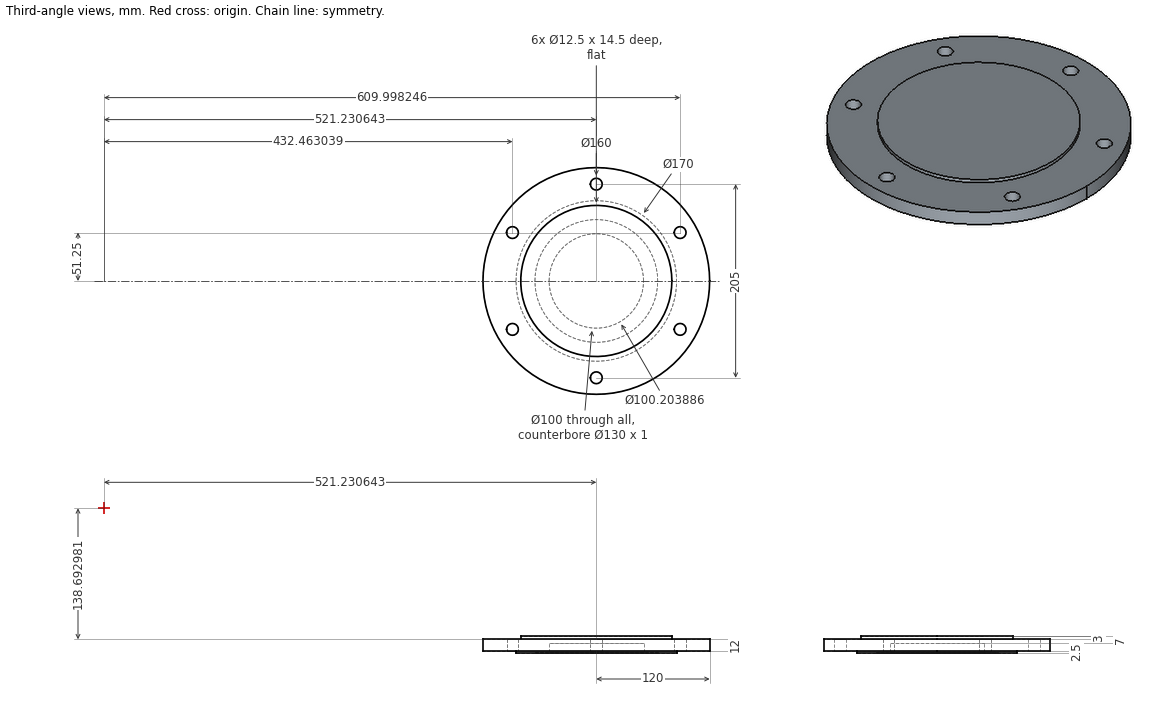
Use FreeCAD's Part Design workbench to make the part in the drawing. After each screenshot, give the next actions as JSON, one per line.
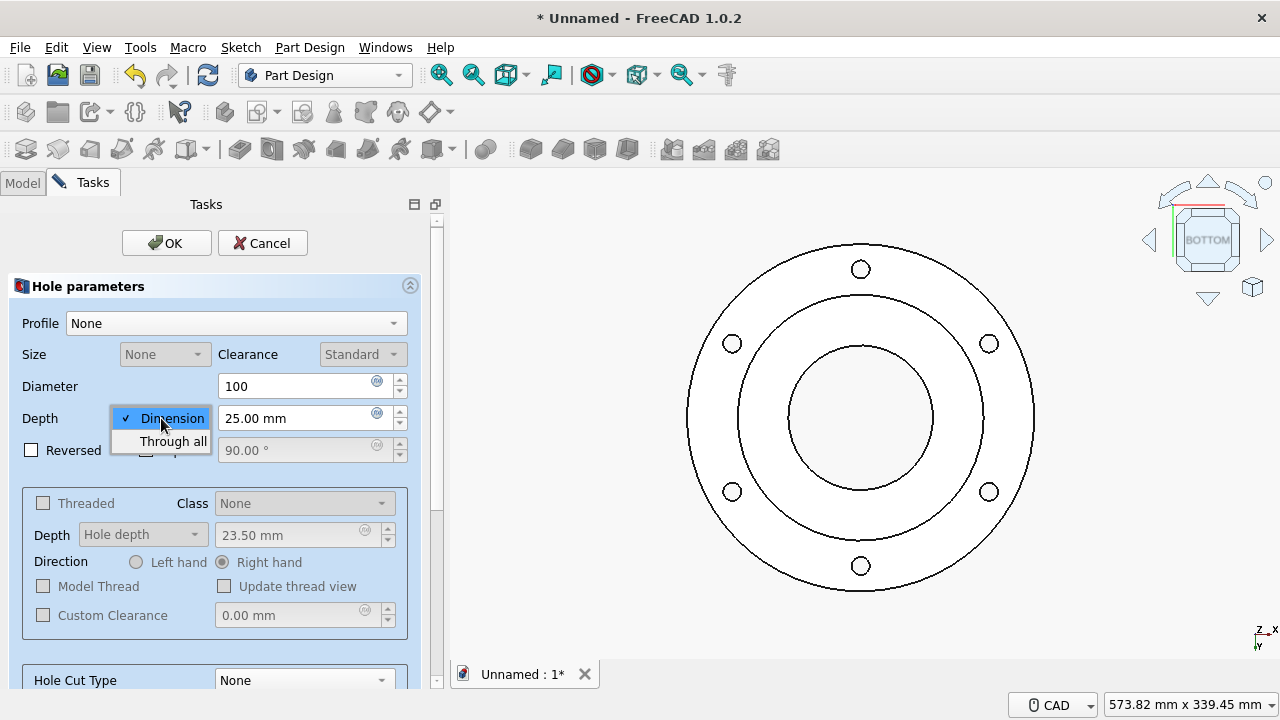
{"action": "left_click", "coordinate": [160, 442]}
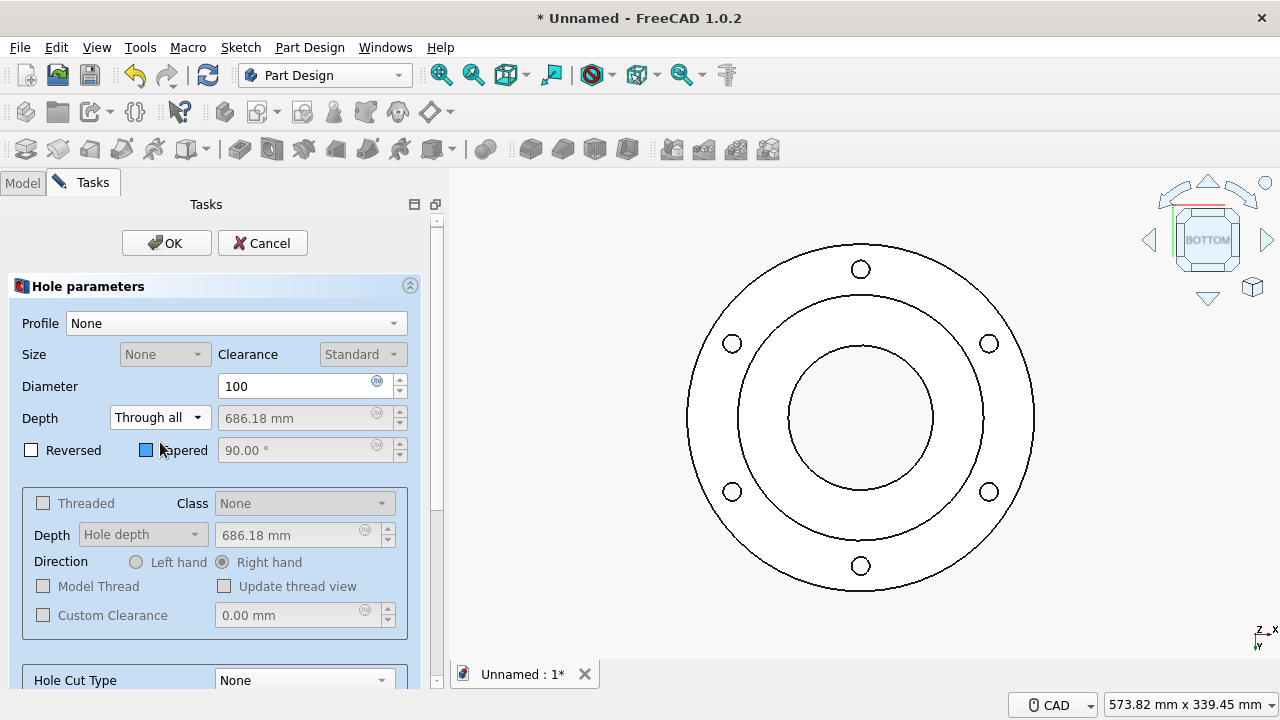
{"action": "scroll", "coordinate": [437, 451], "scroll_direction": "down", "scroll_amount": 2}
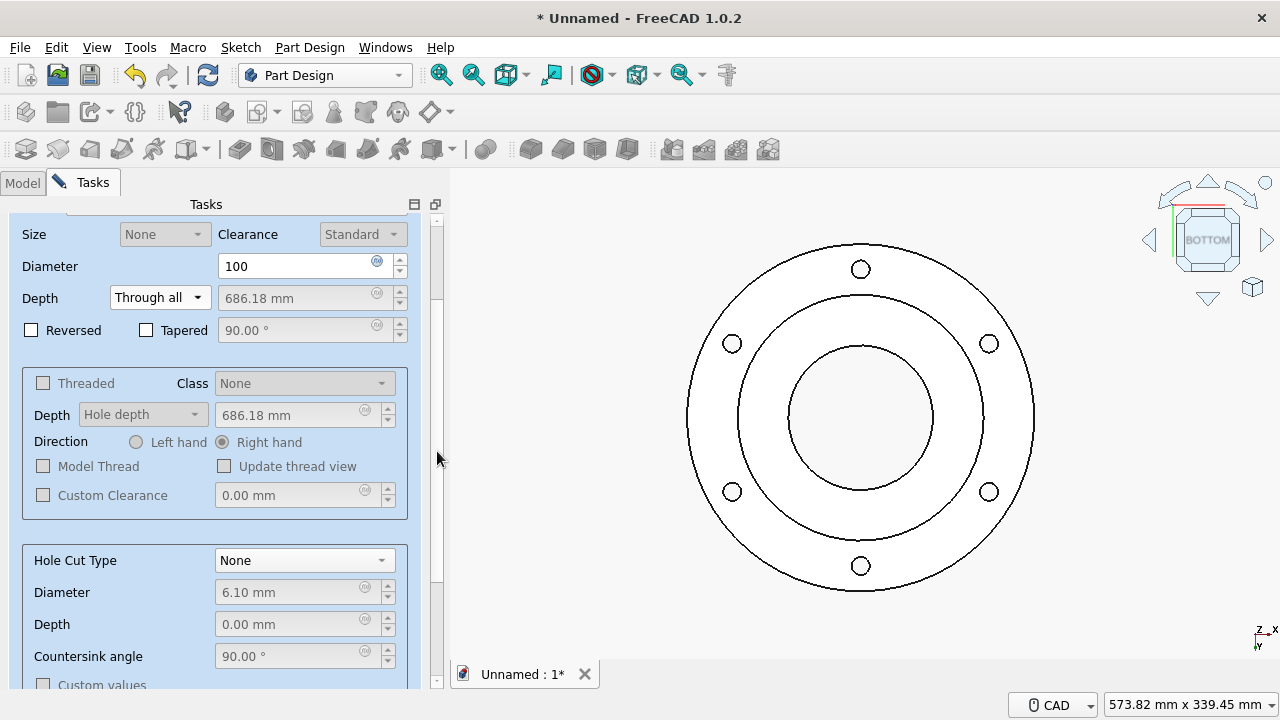
{"action": "left_click", "coordinate": [306, 560]}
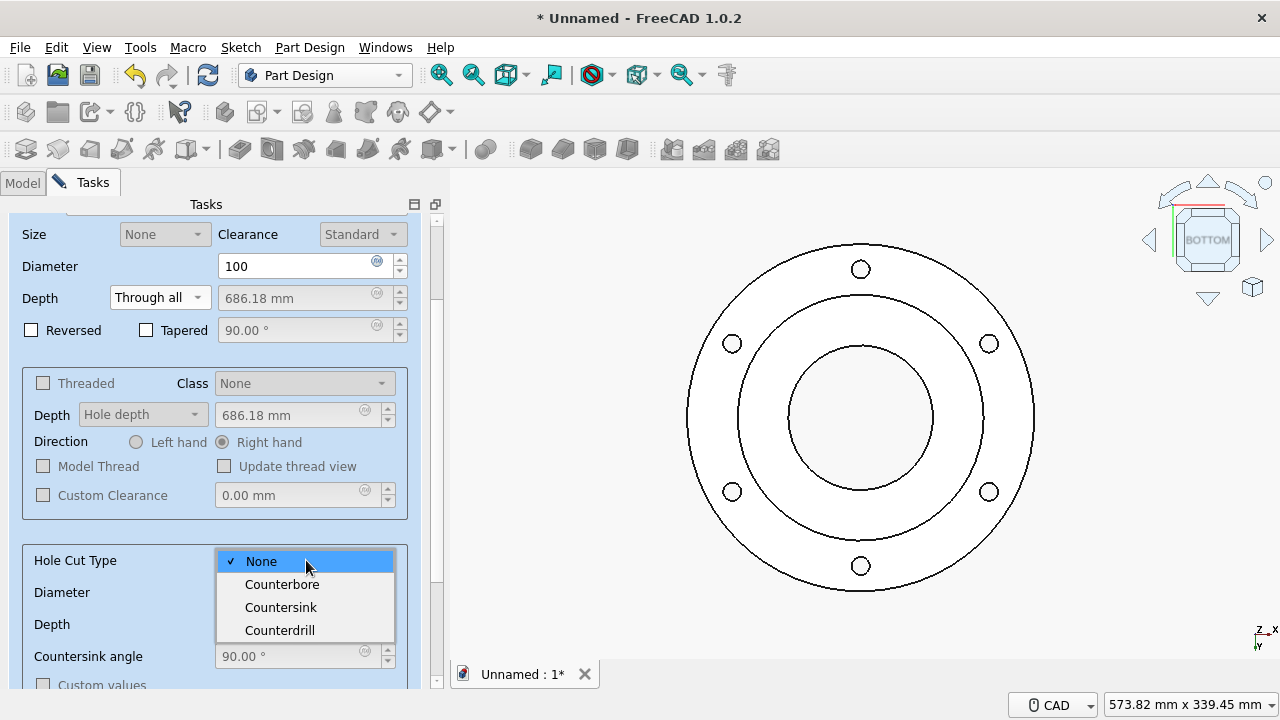
{"action": "left_click", "coordinate": [304, 584]}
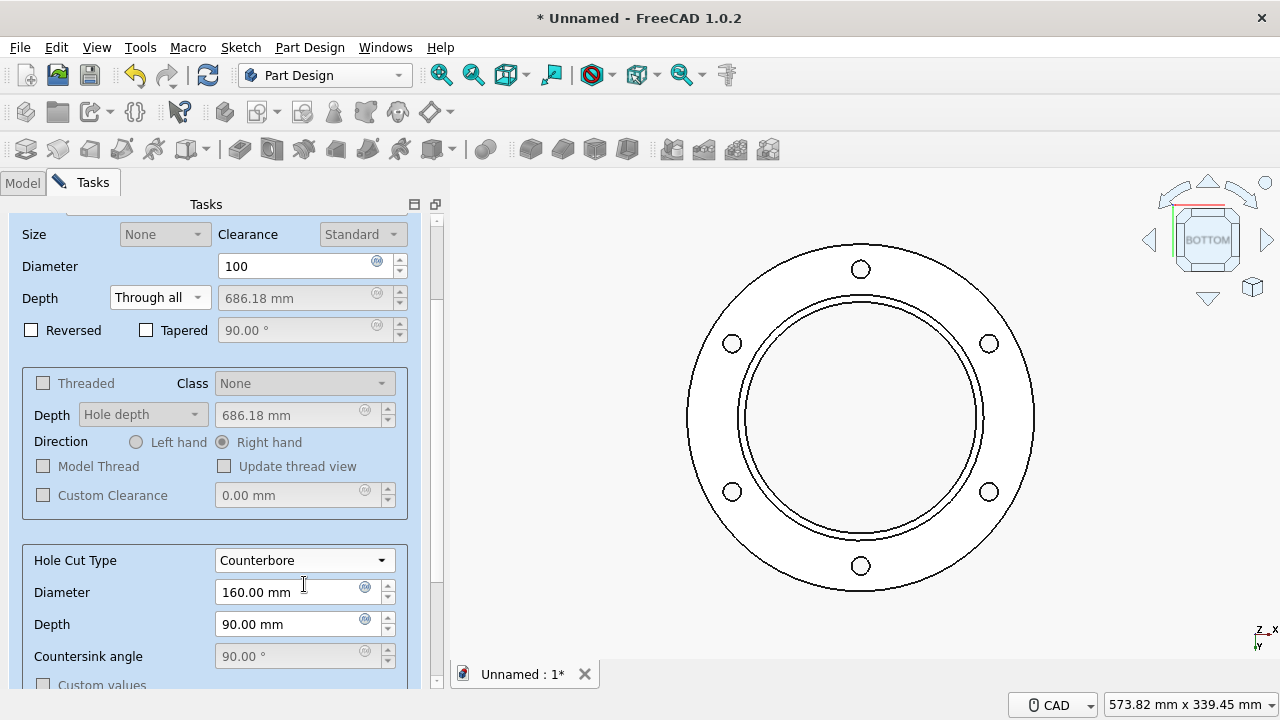
{"action": "triple_click", "coordinate": [298, 592]}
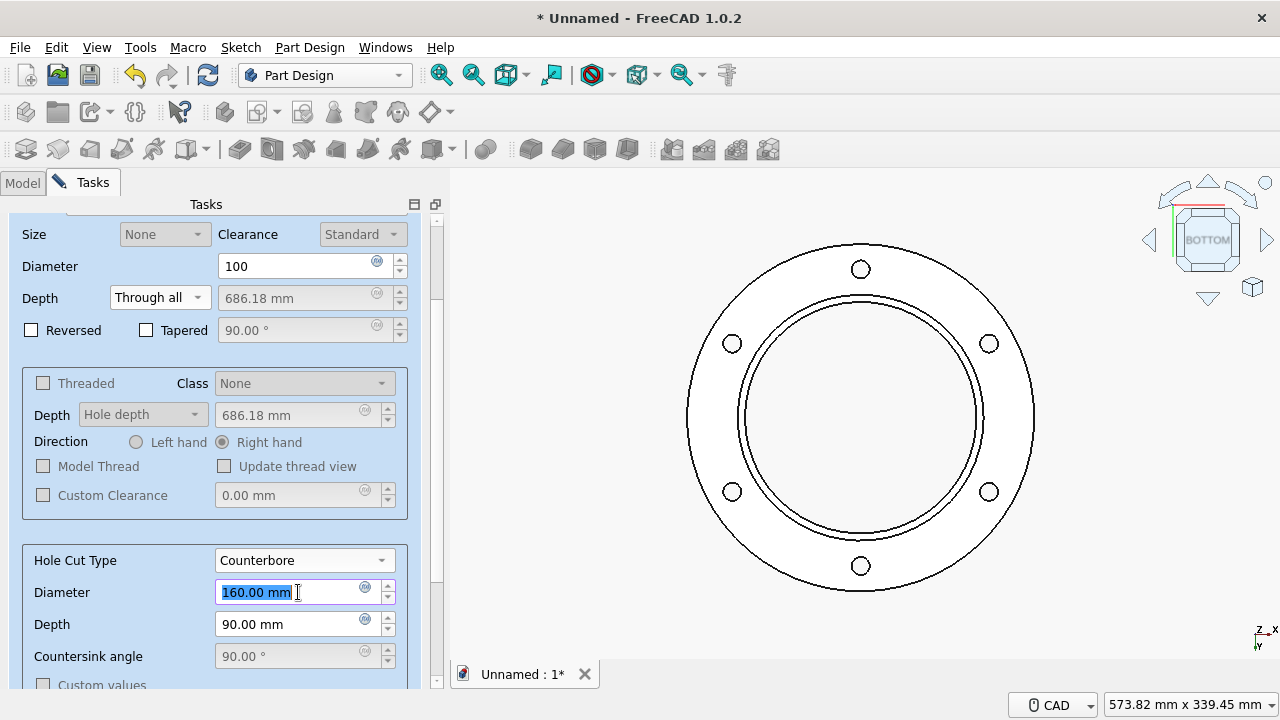
{"action": "type", "text": "130"}
{"action": "key", "text": "Tab"}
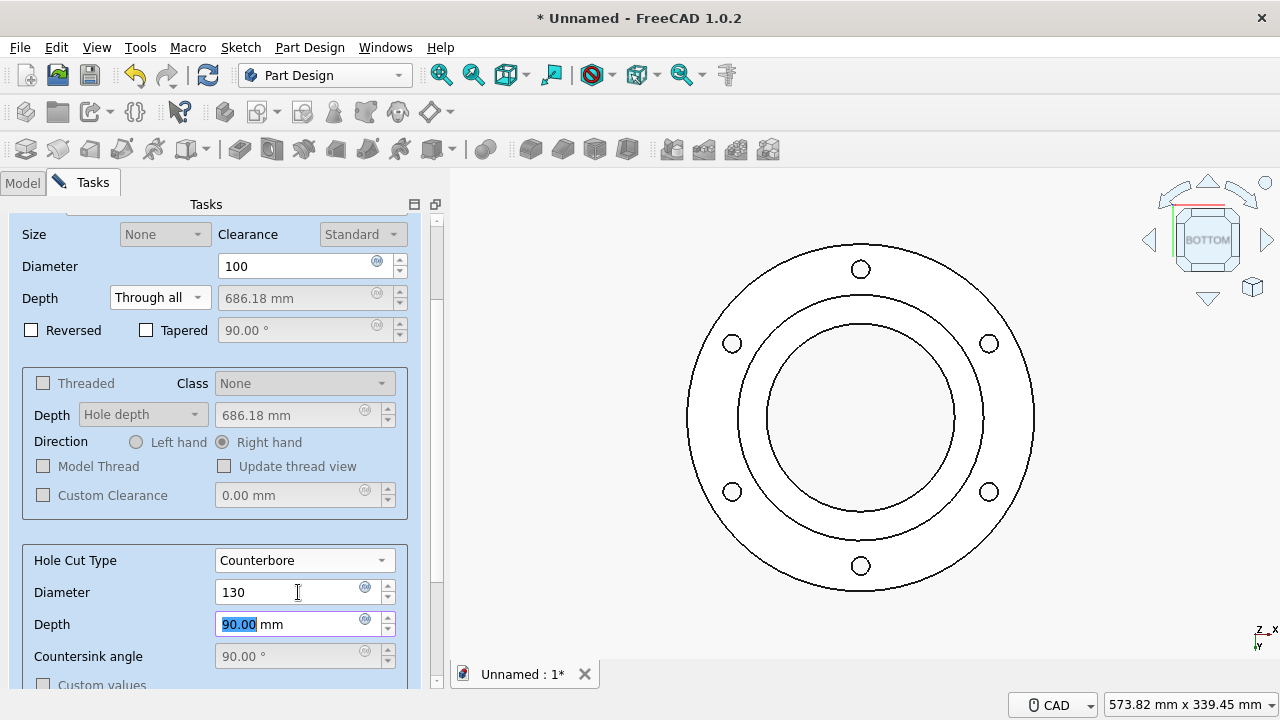
{"action": "type", "text": "1"}
{"action": "key", "text": "Tab"}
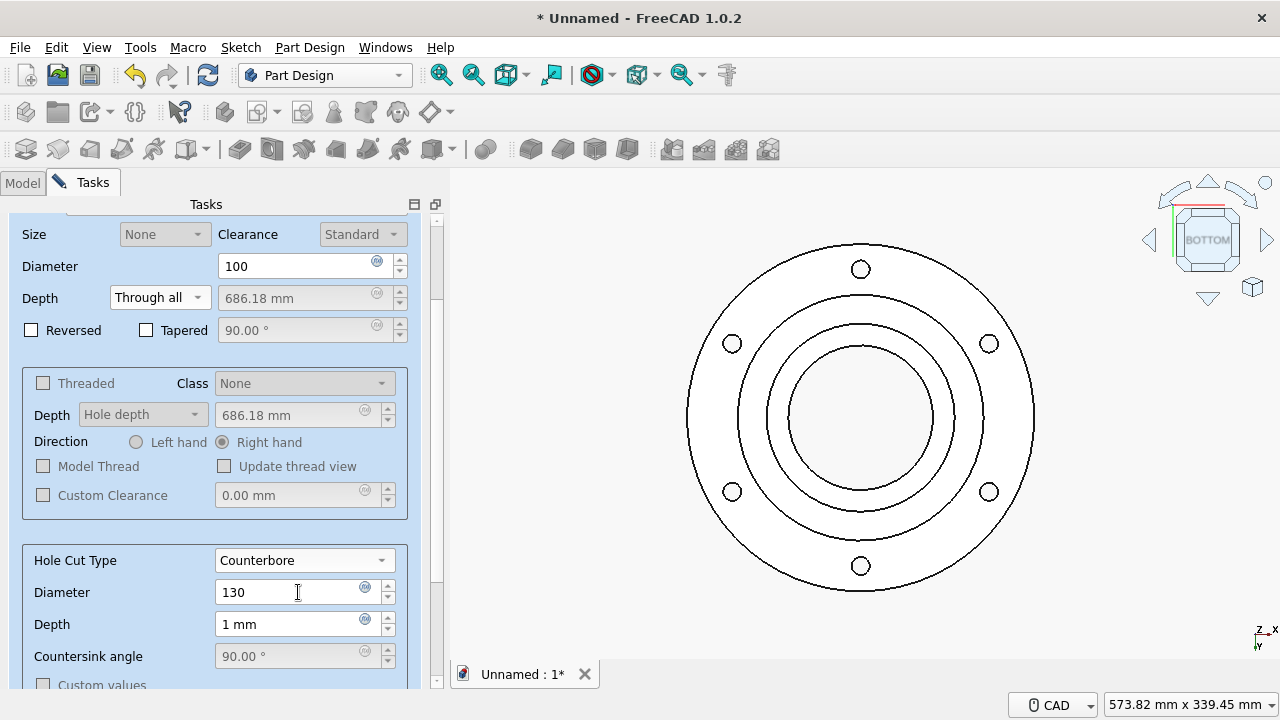
{"action": "scroll", "coordinate": [437, 451], "scroll_direction": "up", "scroll_amount": 3}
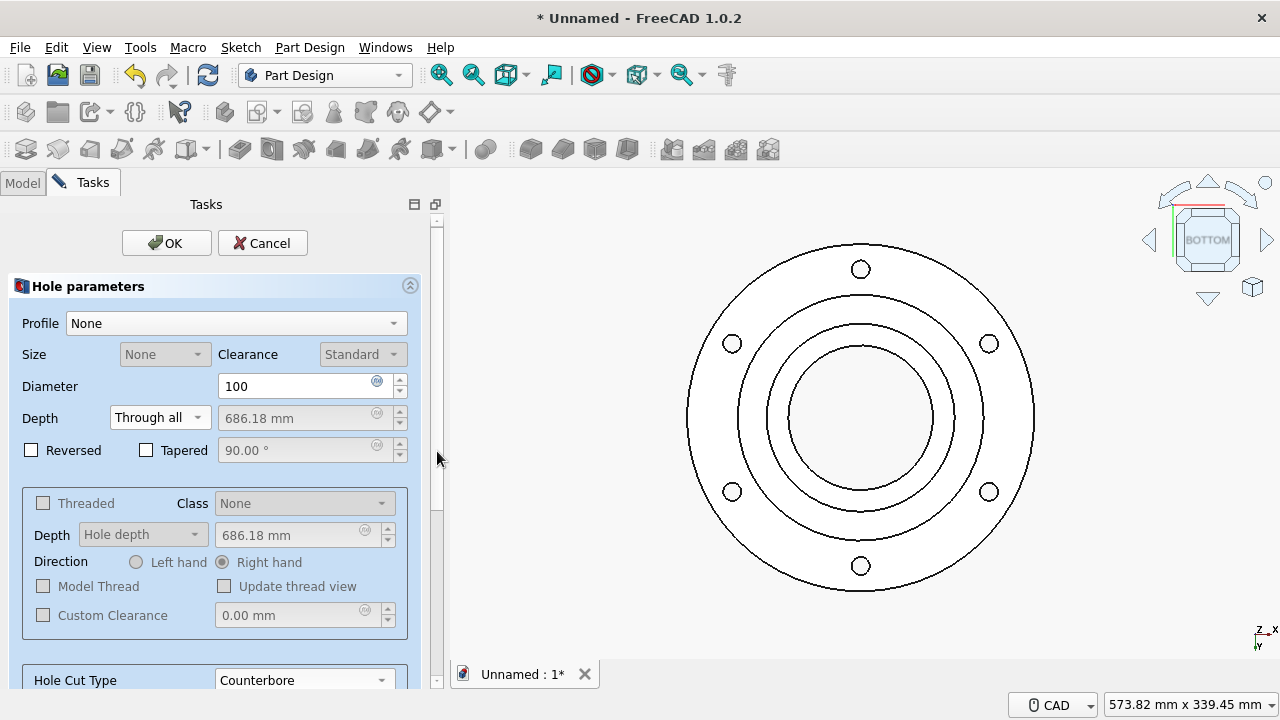
{"action": "left_click", "coordinate": [167, 243]}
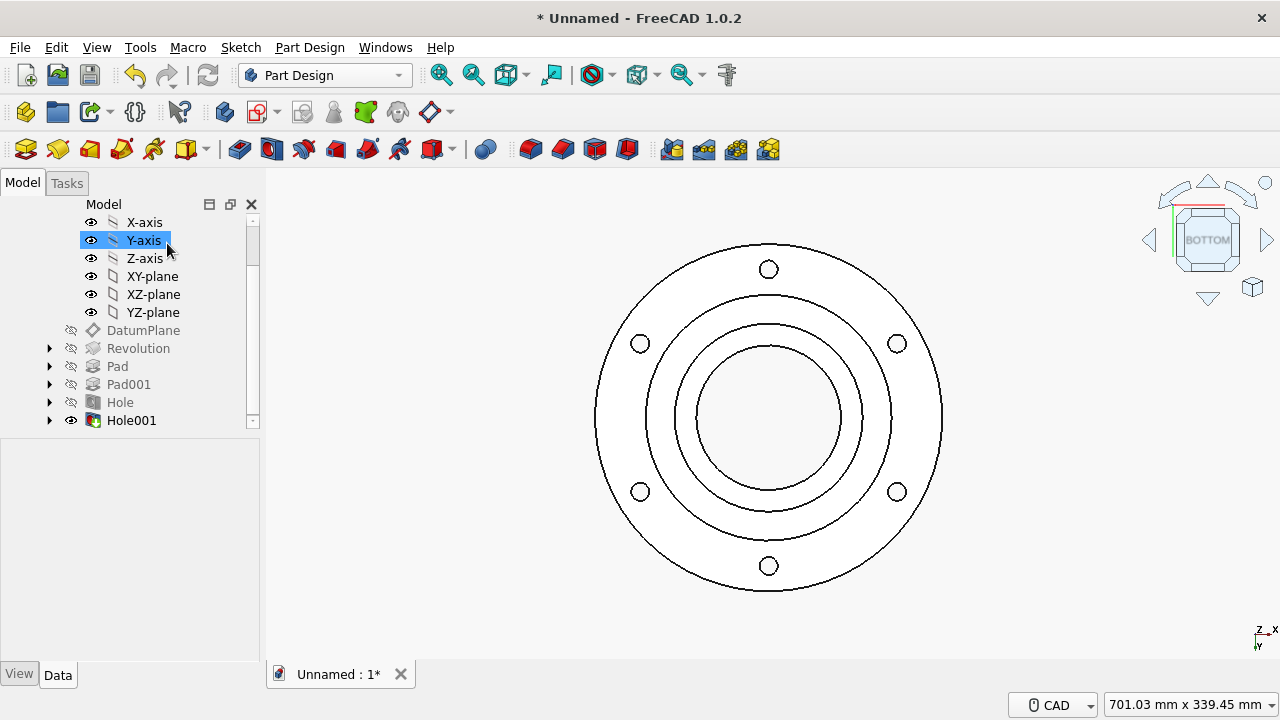
{"action": "key", "text": "0"}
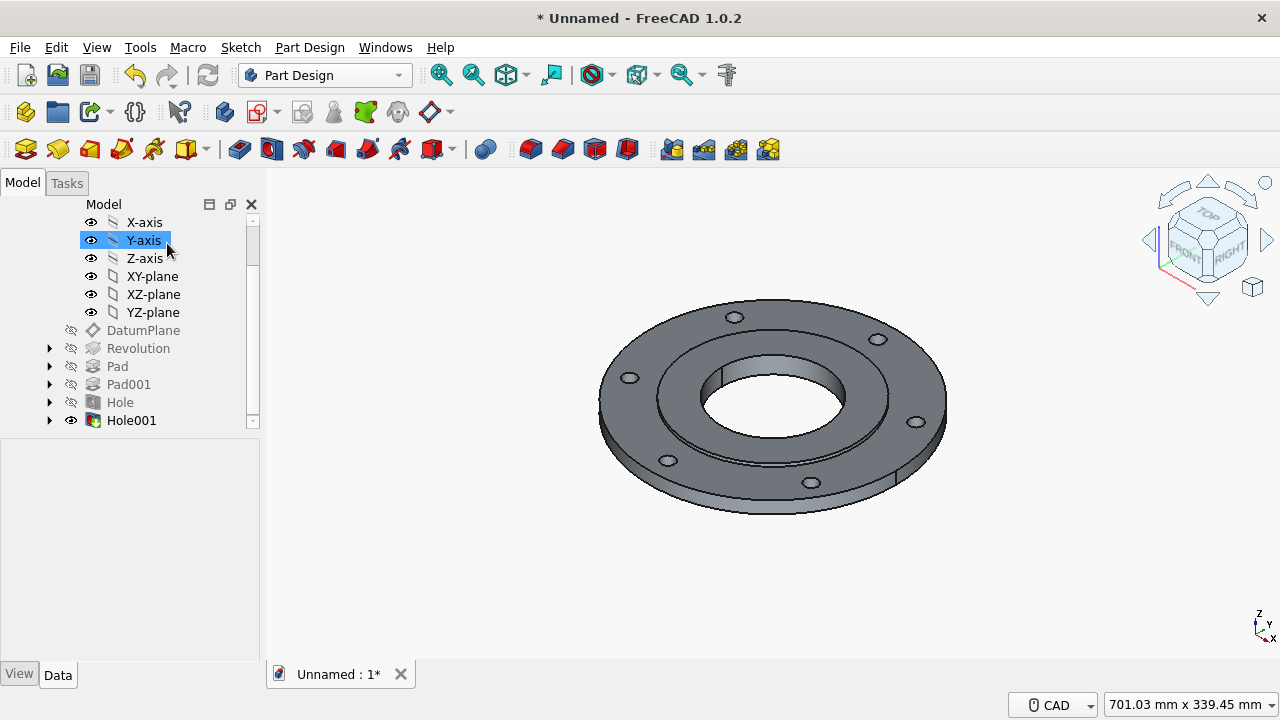
{"action": "left_click", "coordinate": [679, 396]}